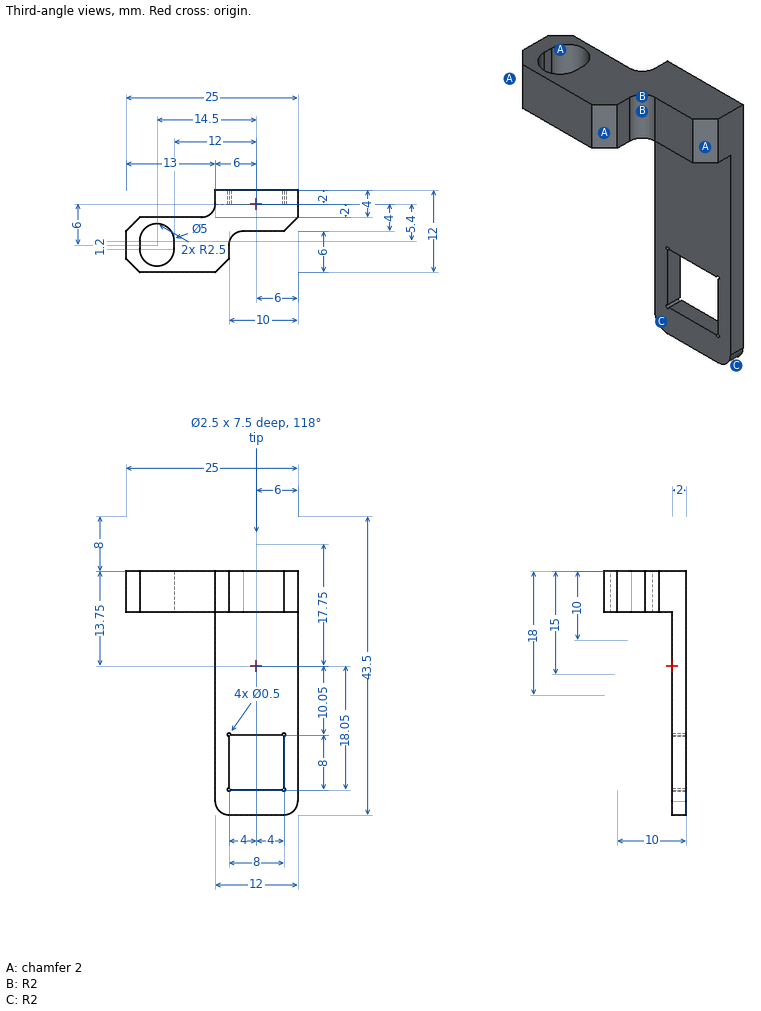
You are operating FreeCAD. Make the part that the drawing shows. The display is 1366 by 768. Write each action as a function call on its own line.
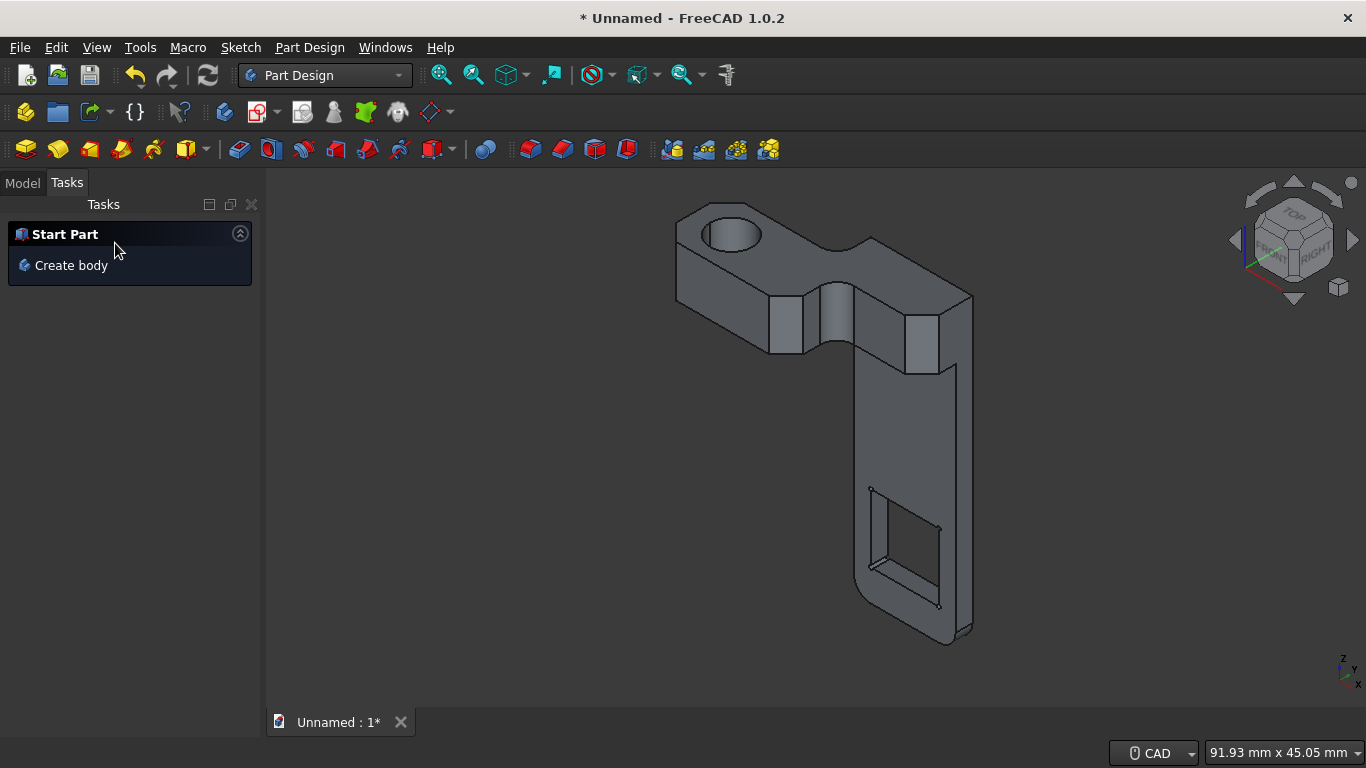
click(905, 281)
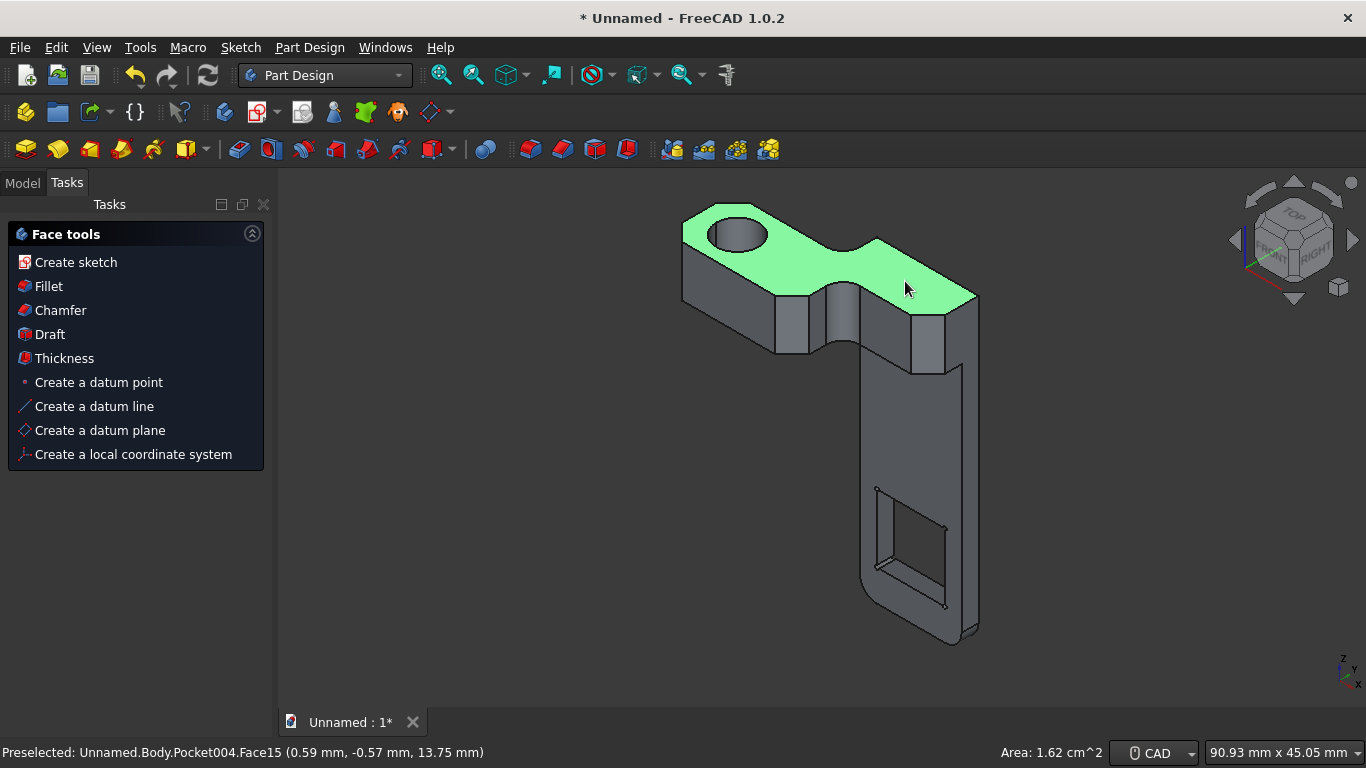
click(258, 112)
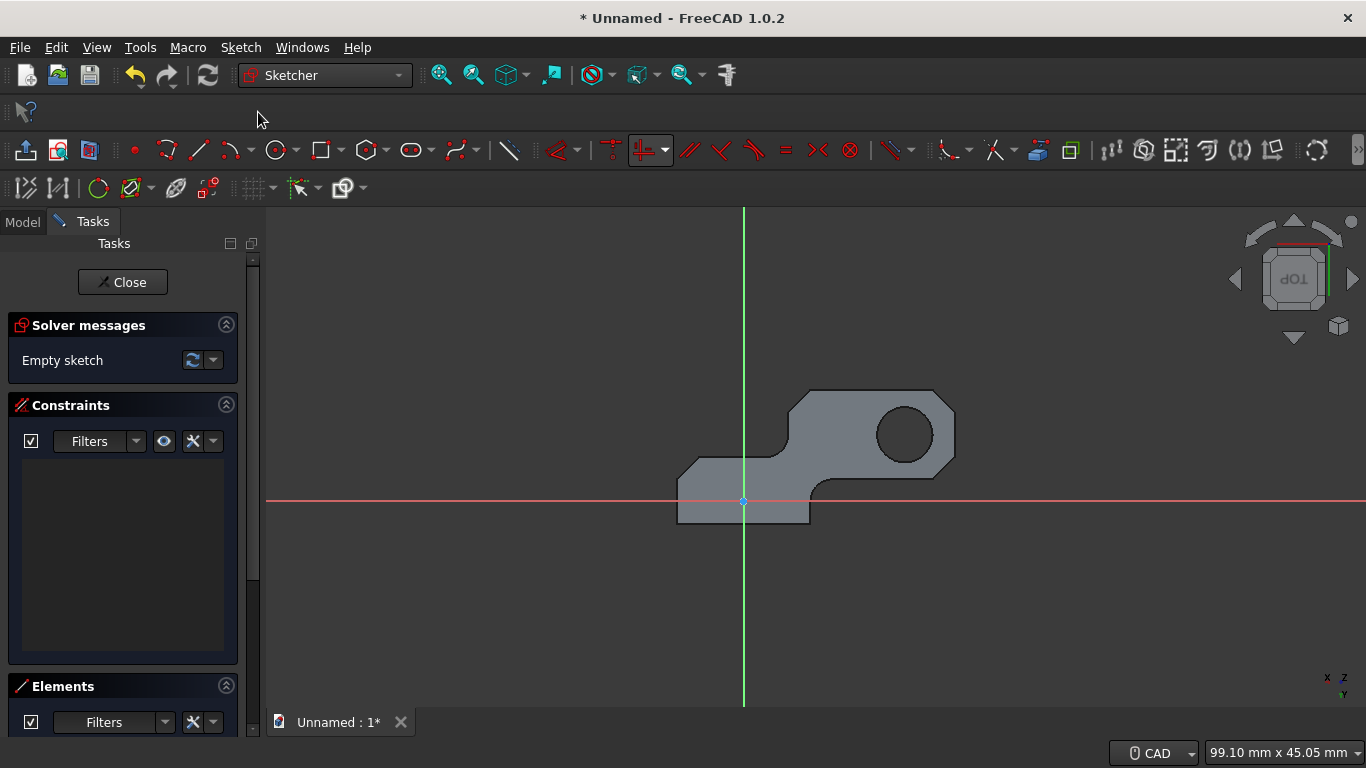
scroll(945, 429, up, 8)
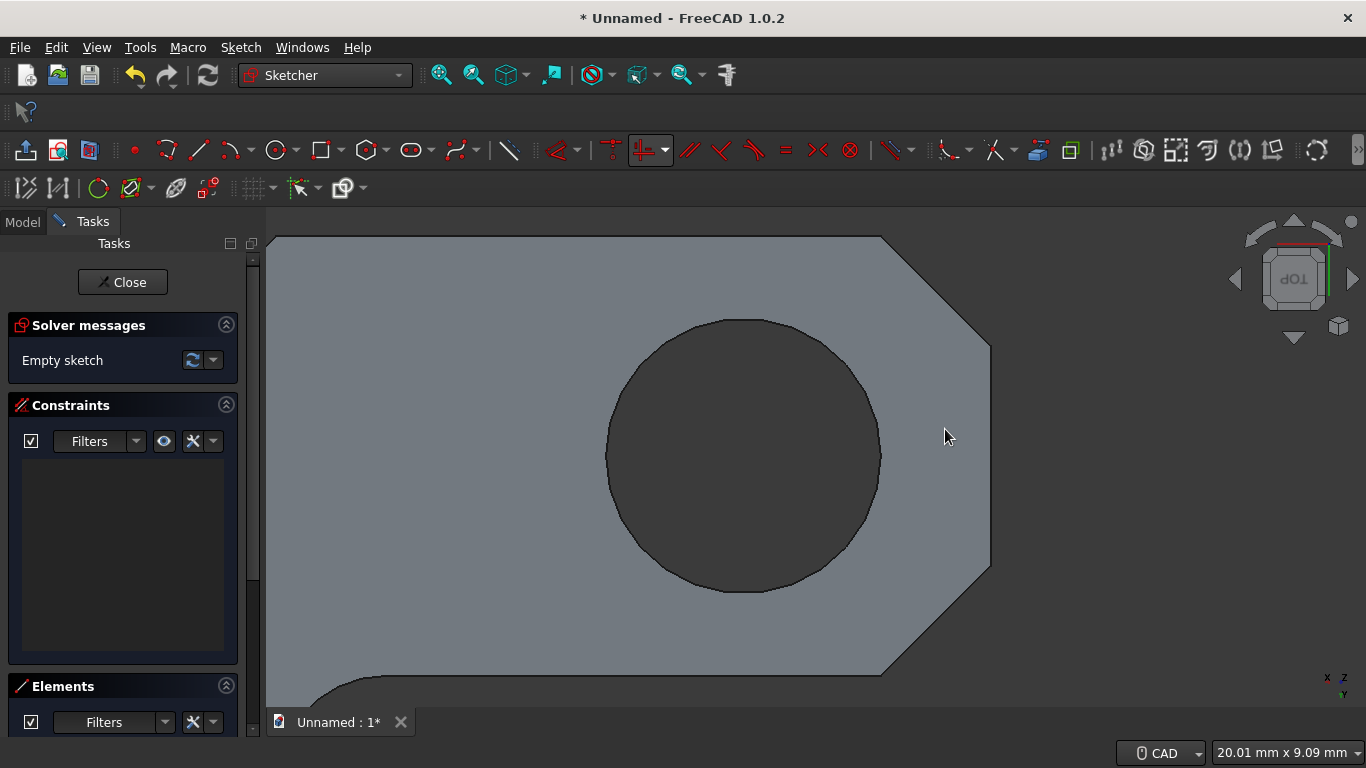
click(412, 150)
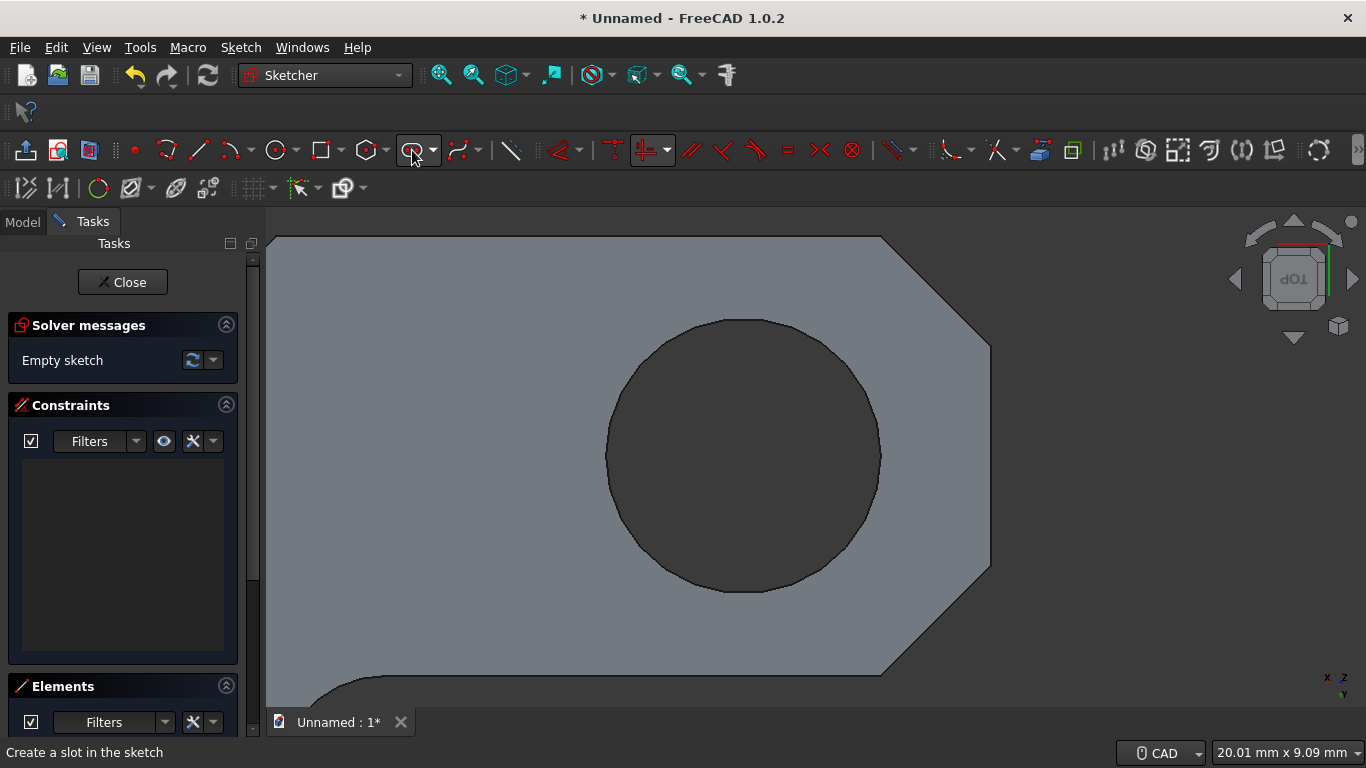
click(743, 489)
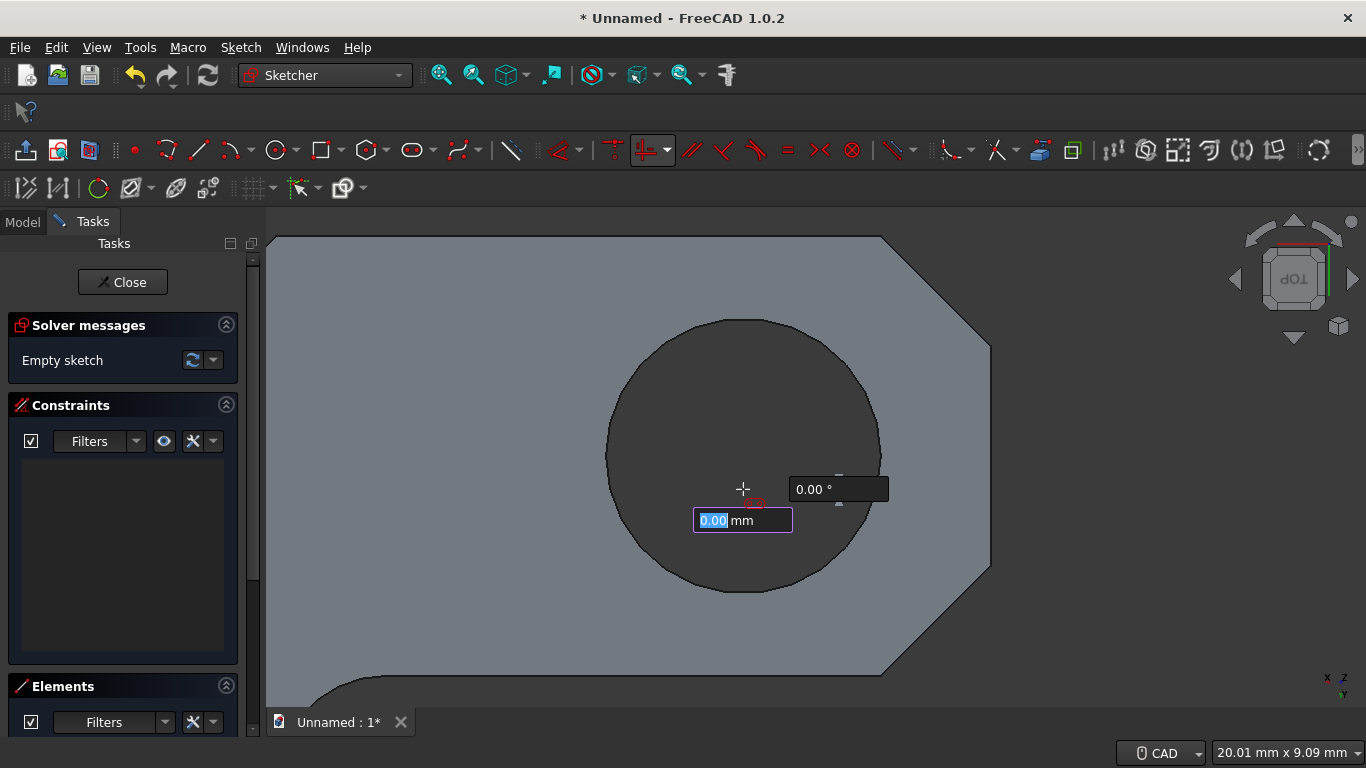
click(743, 423)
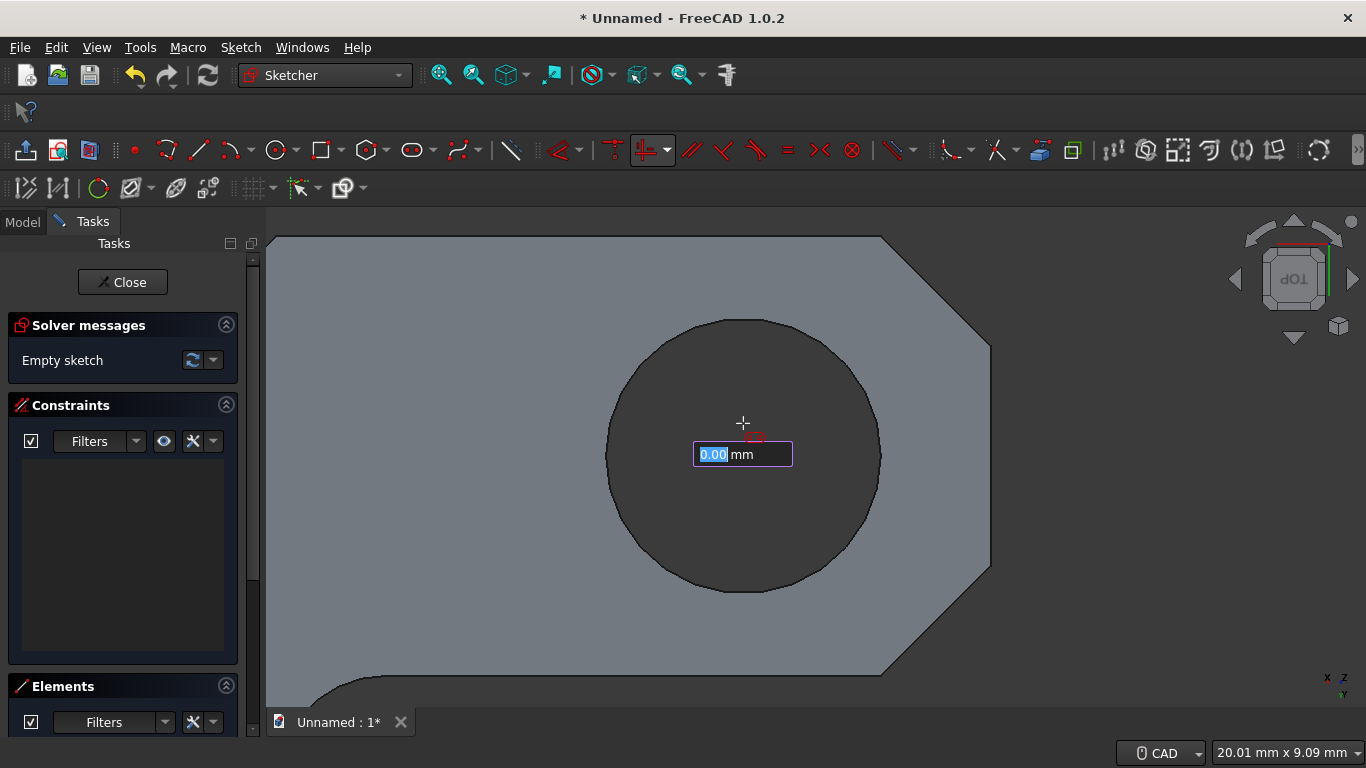
click(606, 456)
key(Escape)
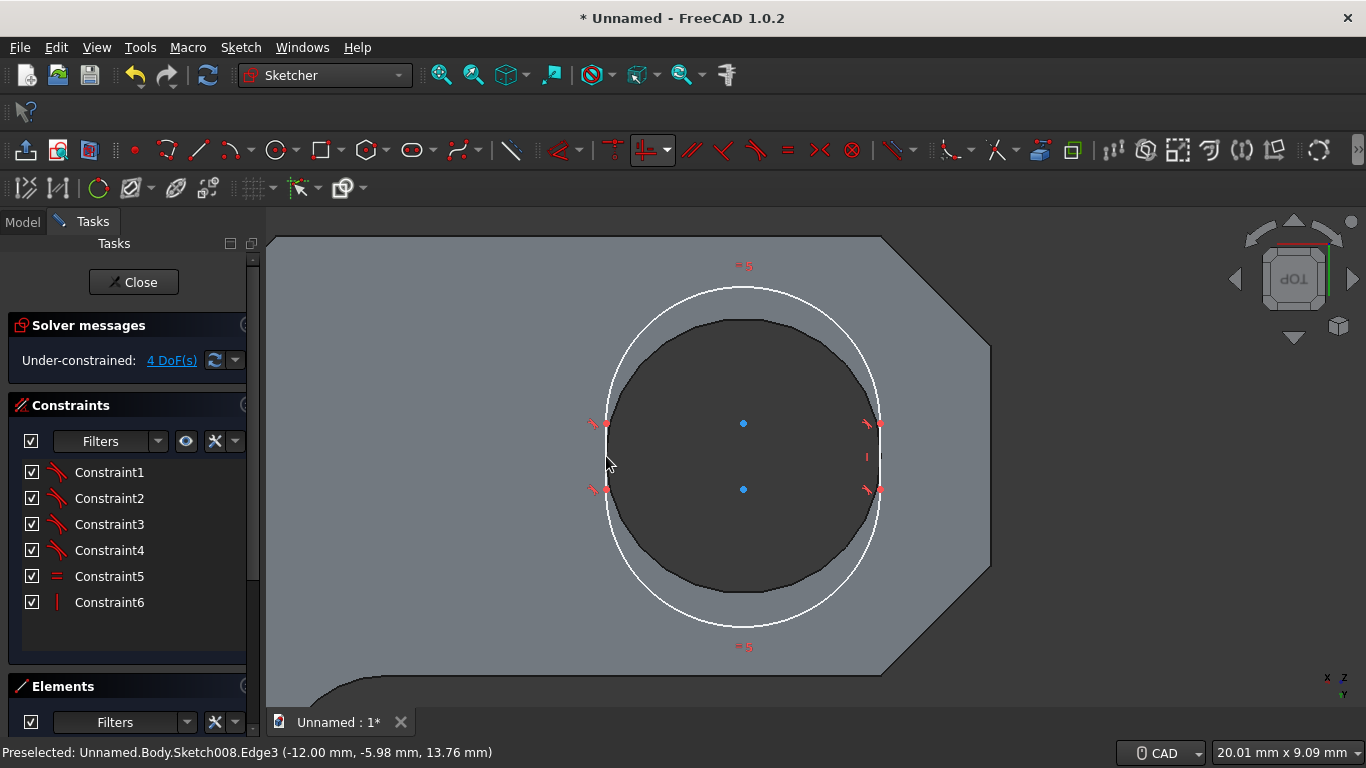
click(558, 150)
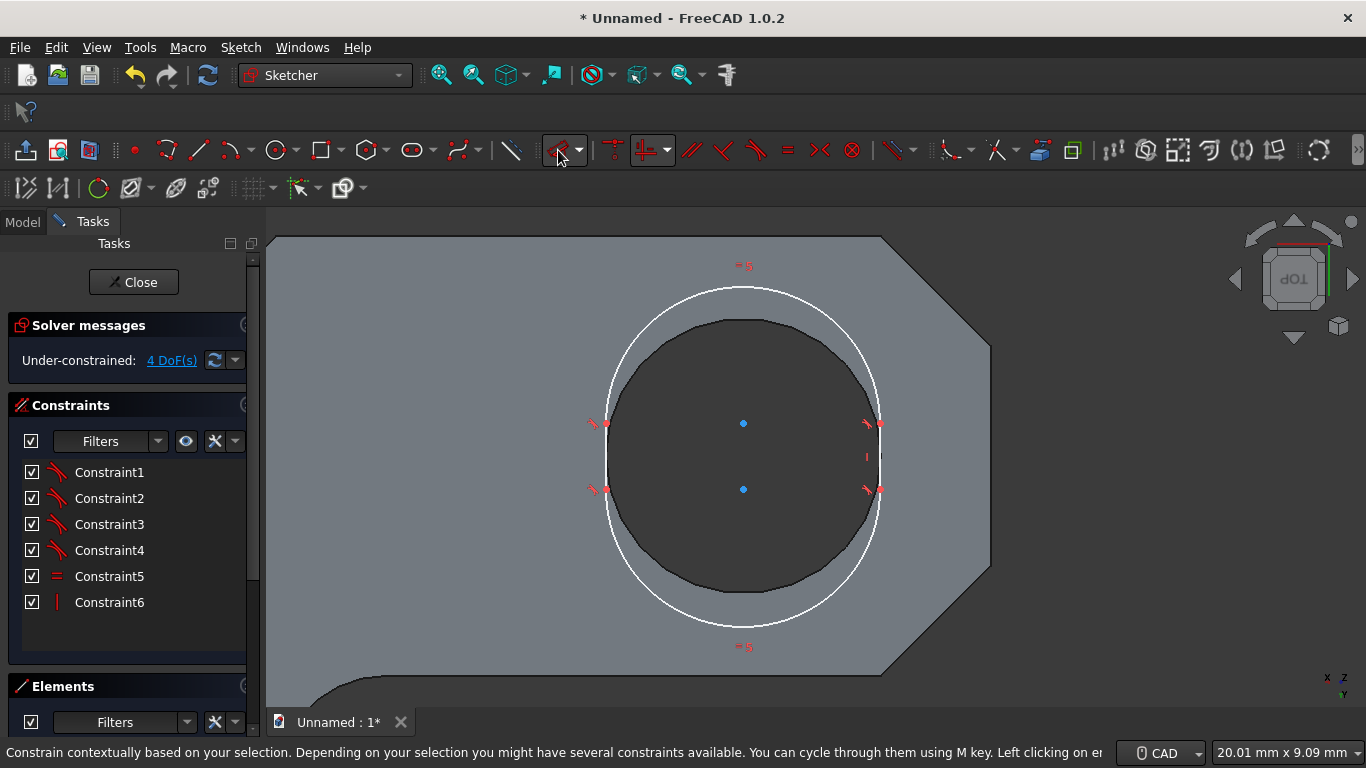
click(662, 601)
click(643, 627)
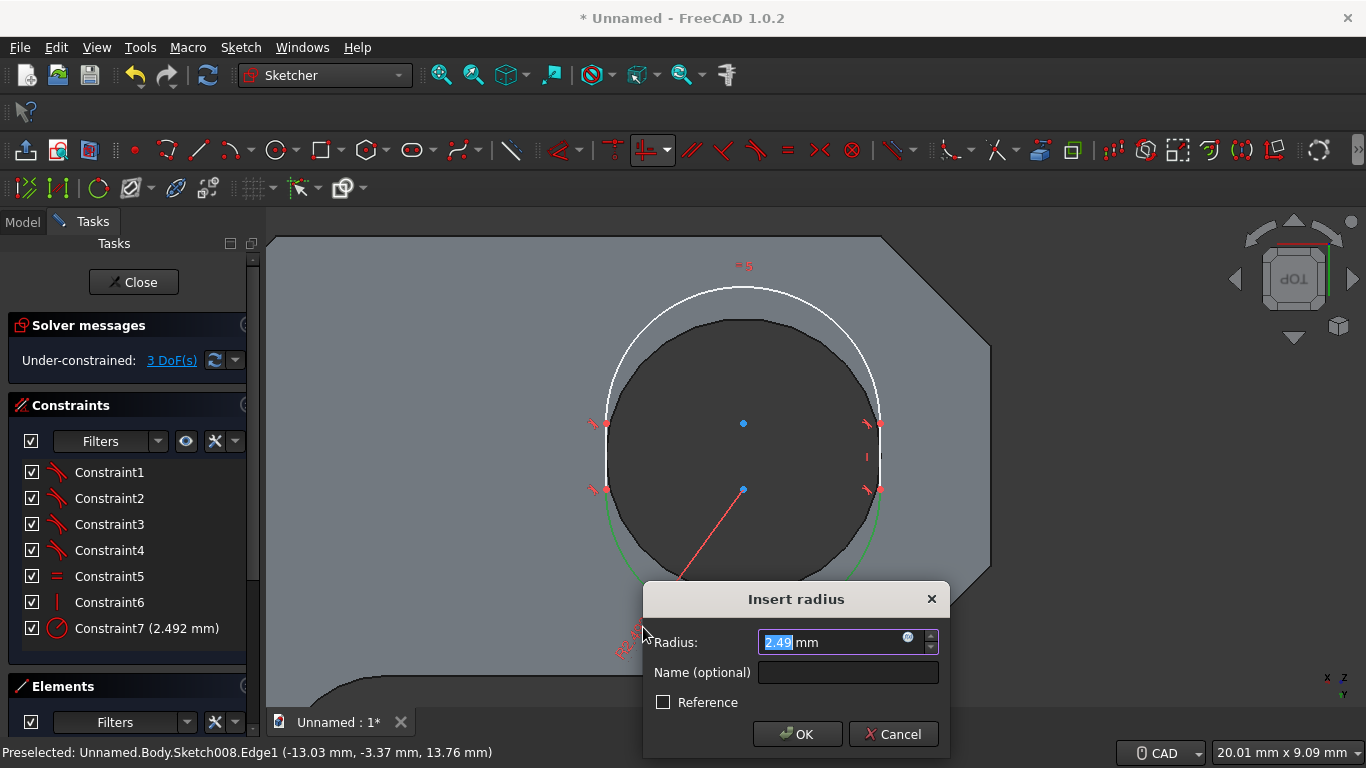
text(2.5)
key(Return)